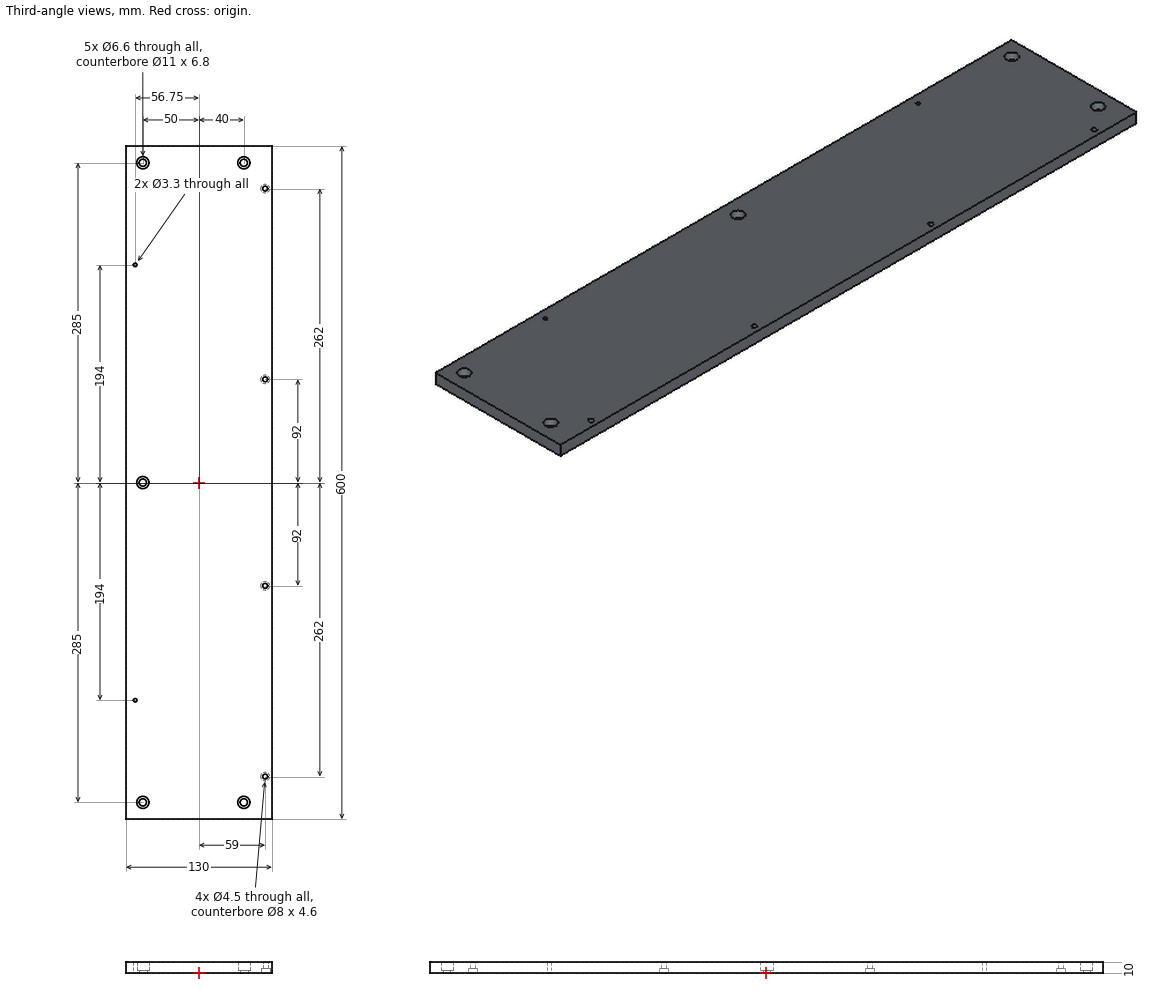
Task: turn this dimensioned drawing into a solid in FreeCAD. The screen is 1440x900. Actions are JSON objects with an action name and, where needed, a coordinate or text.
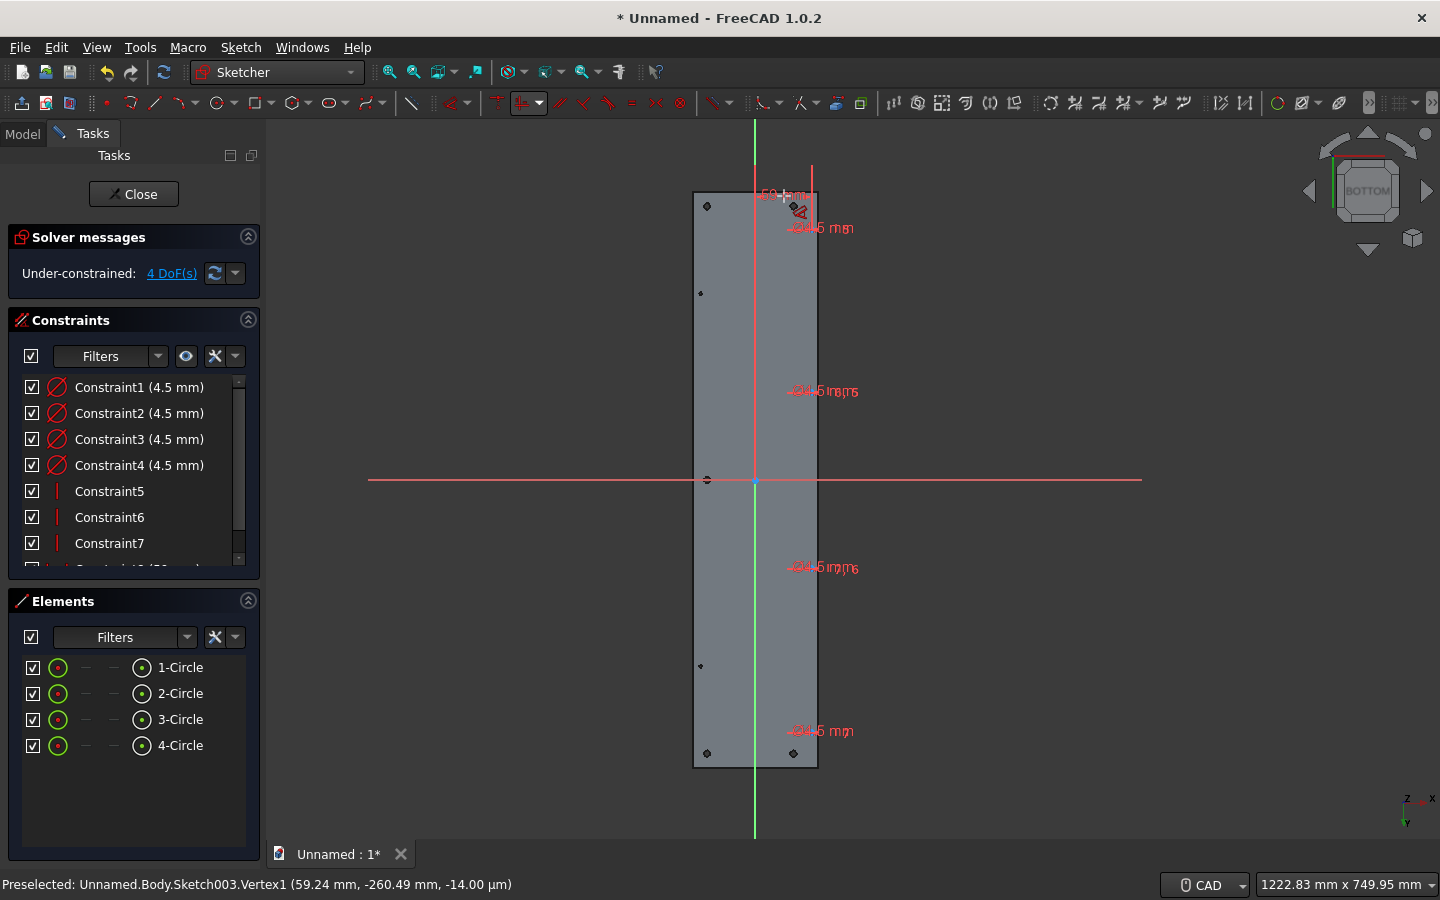
{"action": "left_click", "coordinate": [812, 393]}
{"action": "left_click", "coordinate": [721, 436]}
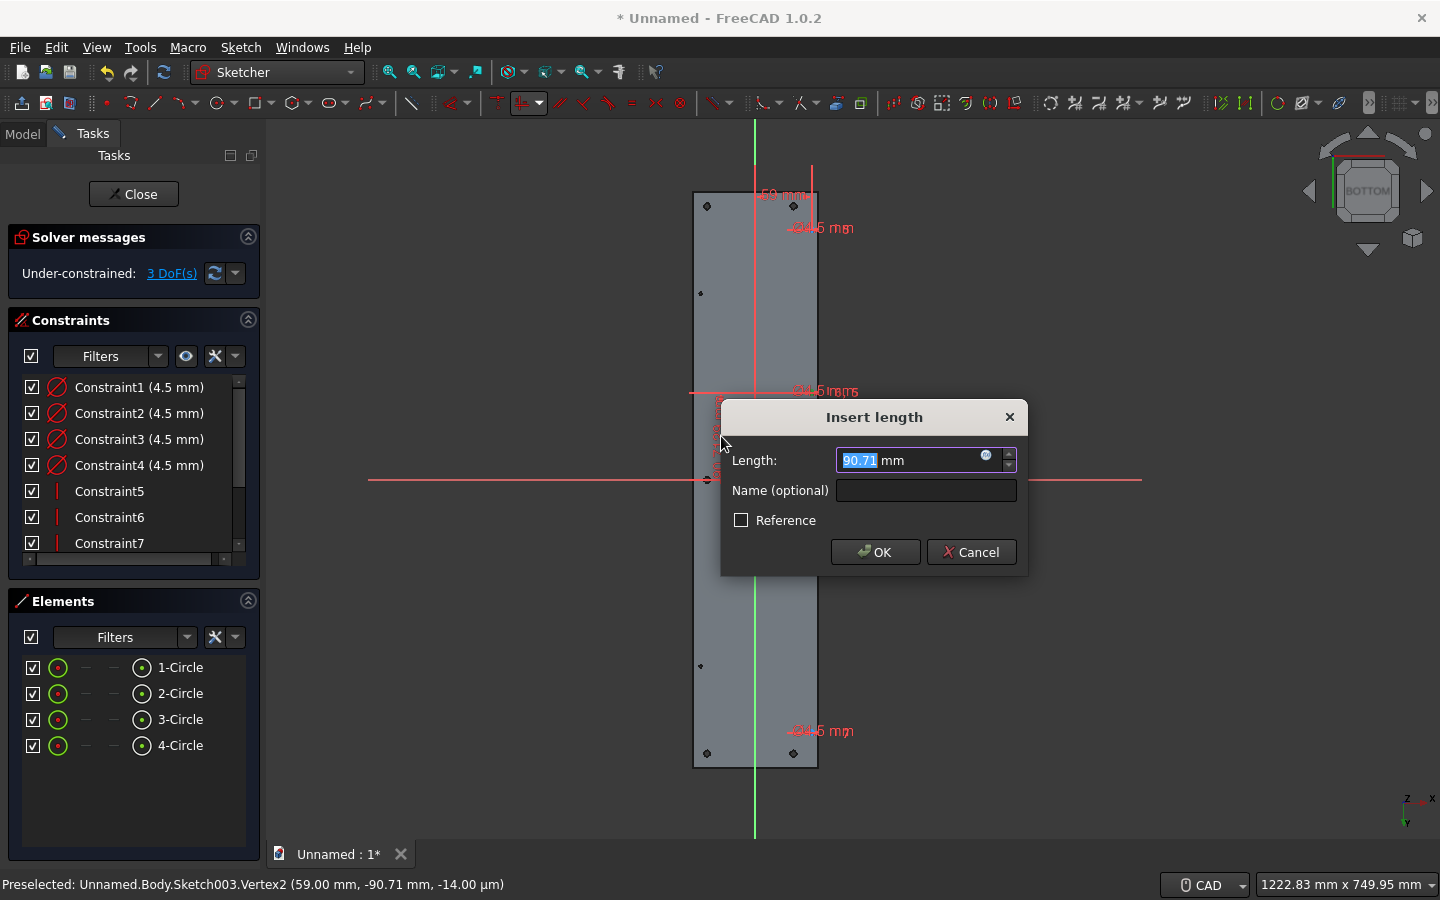
{"action": "type", "text": "92"}
{"action": "key", "text": "Return"}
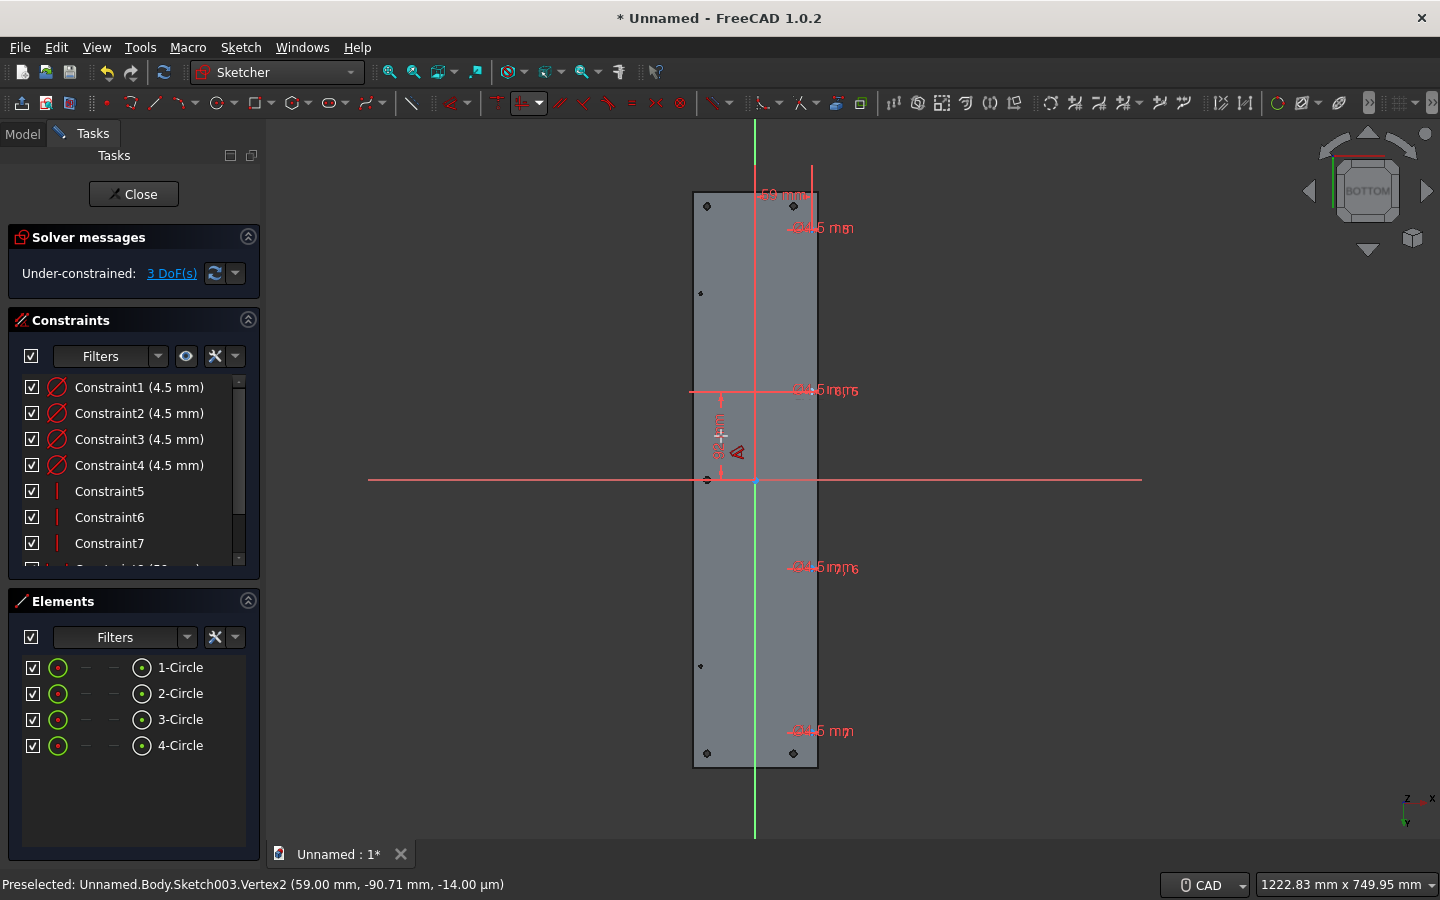
{"action": "left_click", "coordinate": [812, 569]}
{"action": "left_click", "coordinate": [721, 525]}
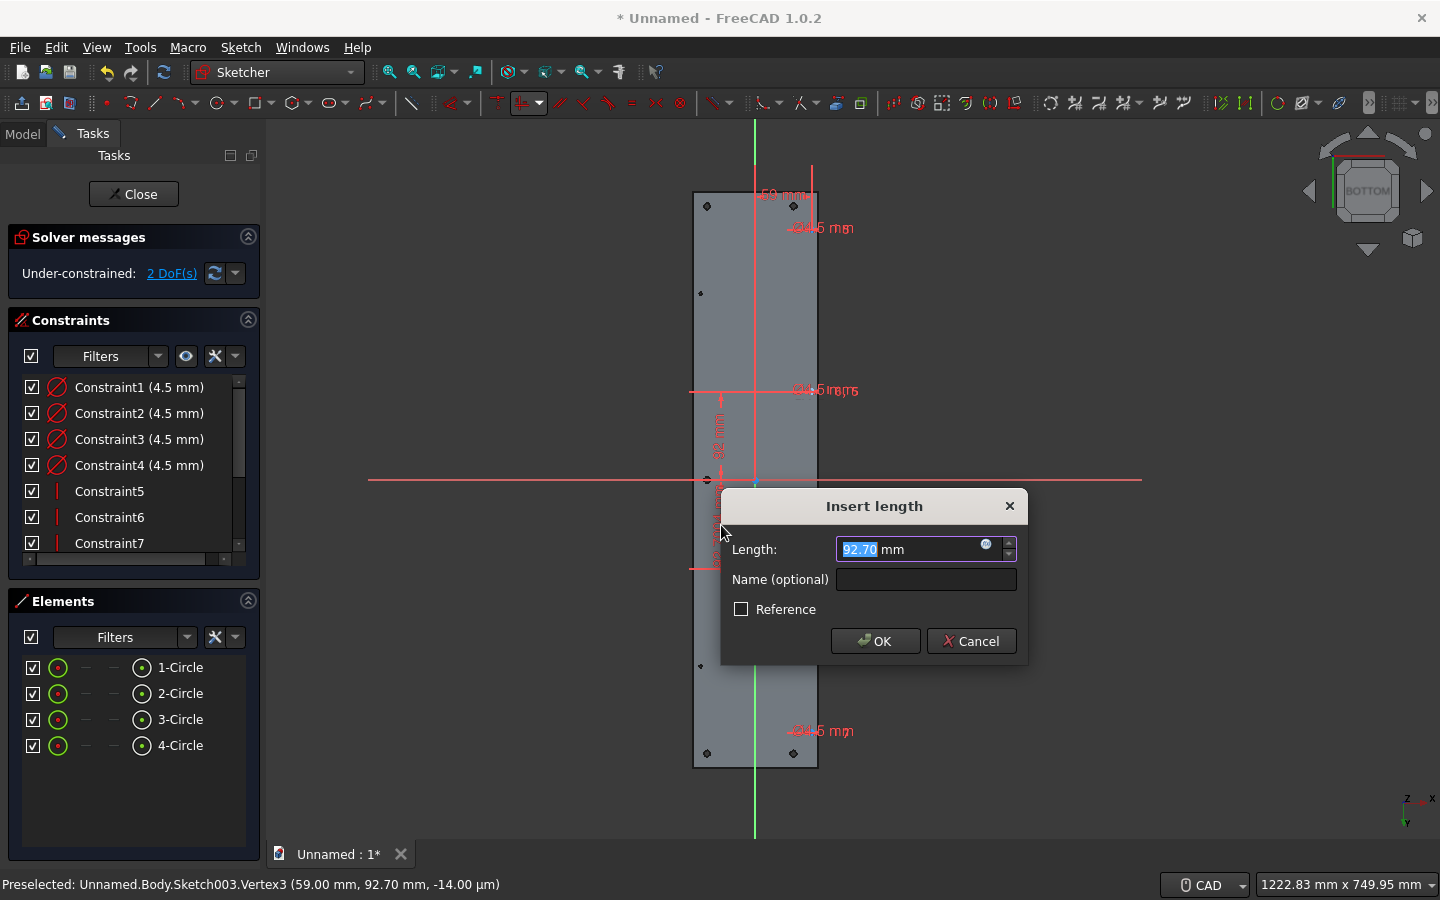
{"action": "type", "text": "92"}
{"action": "key", "text": "Return"}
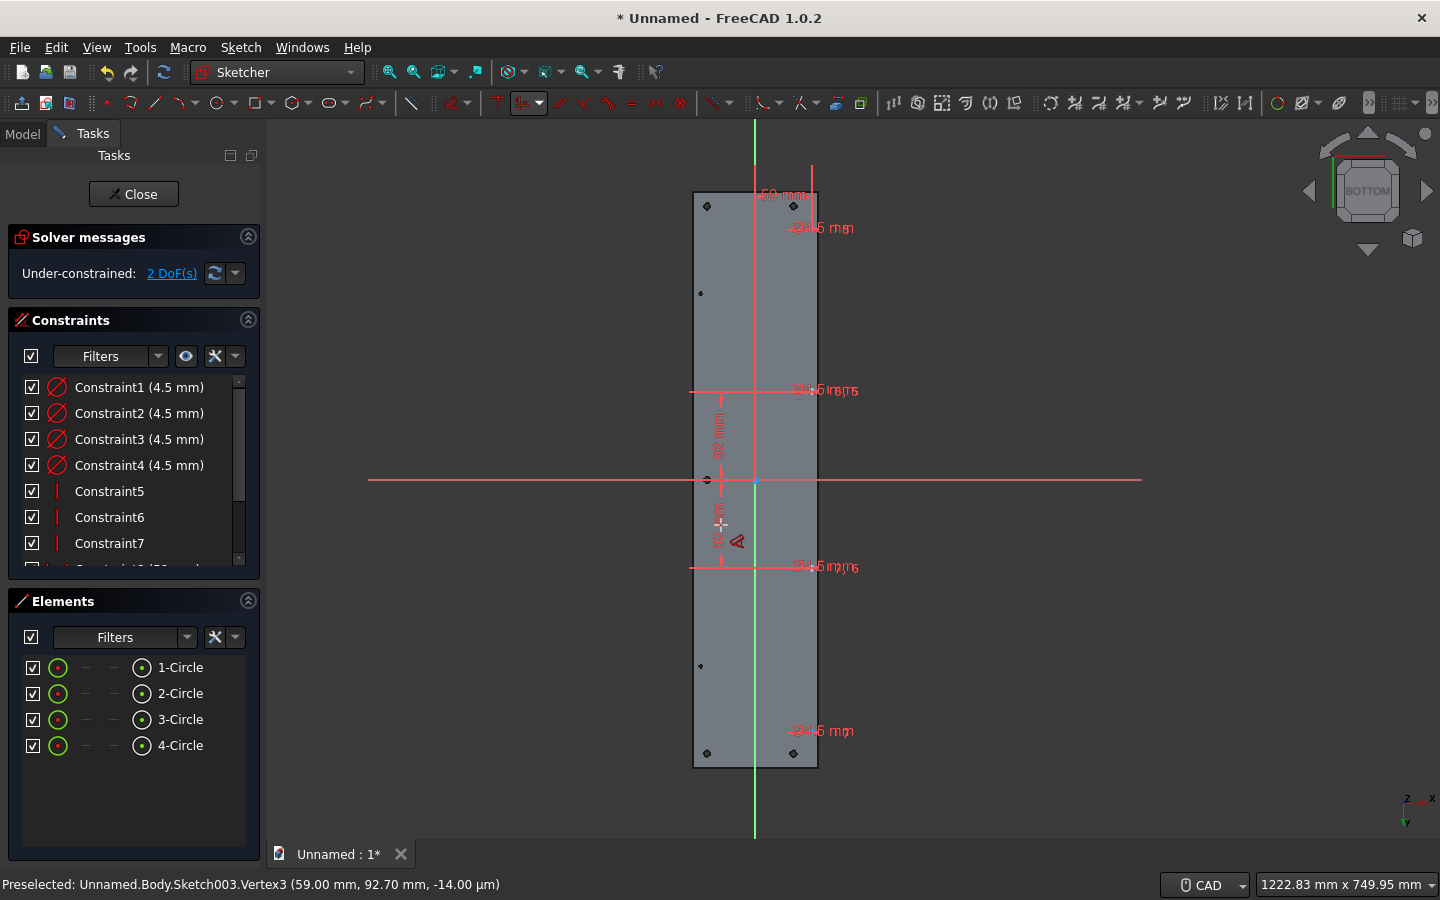
{"action": "left_click", "coordinate": [812, 230]}
{"action": "left_click", "coordinate": [721, 355]}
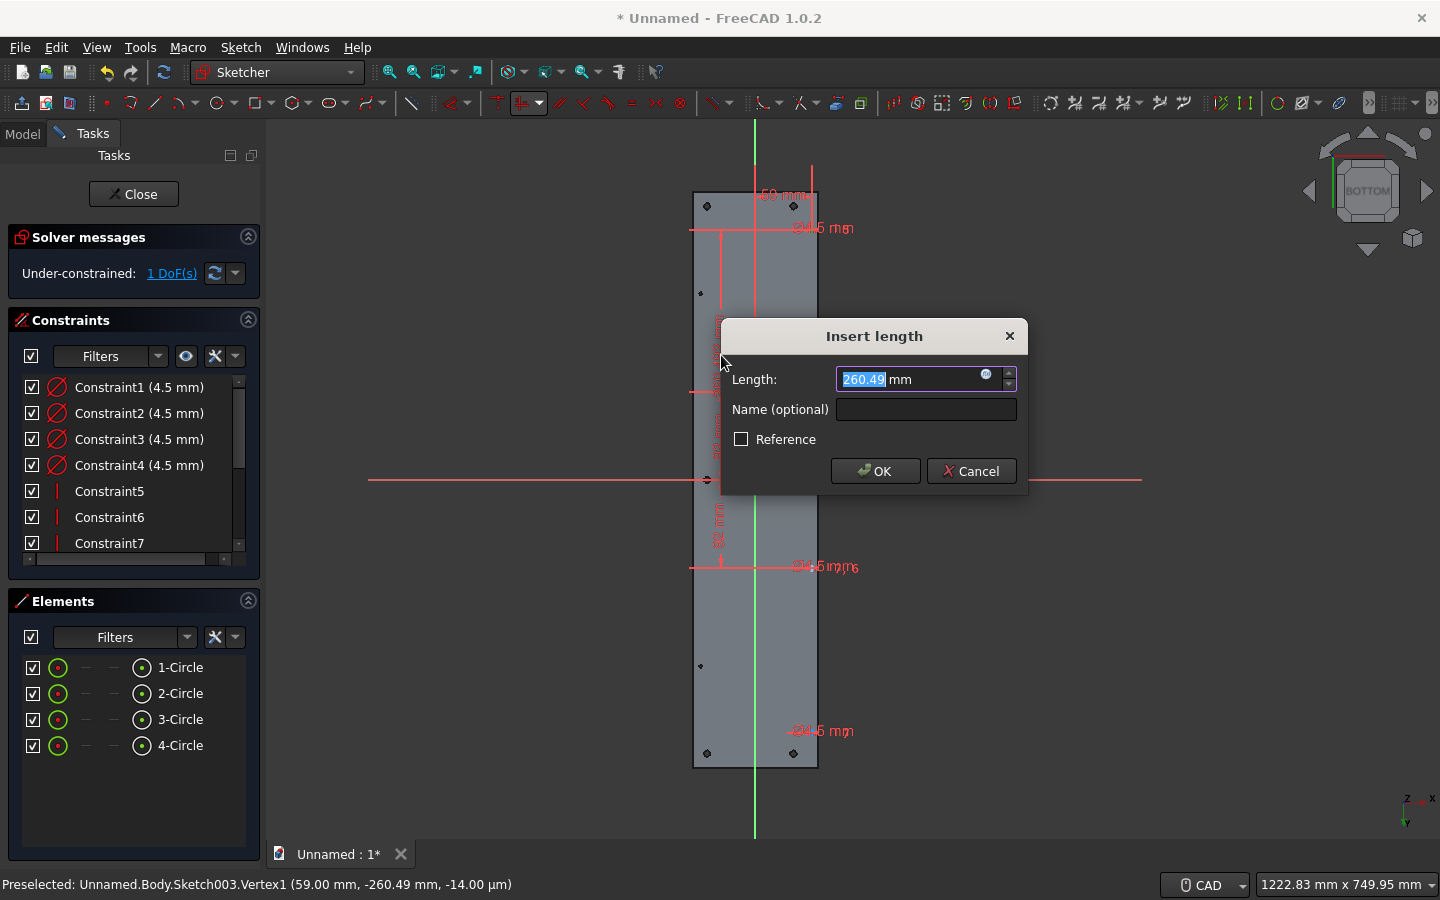
{"action": "type", "text": "262"}
{"action": "key", "text": "Return"}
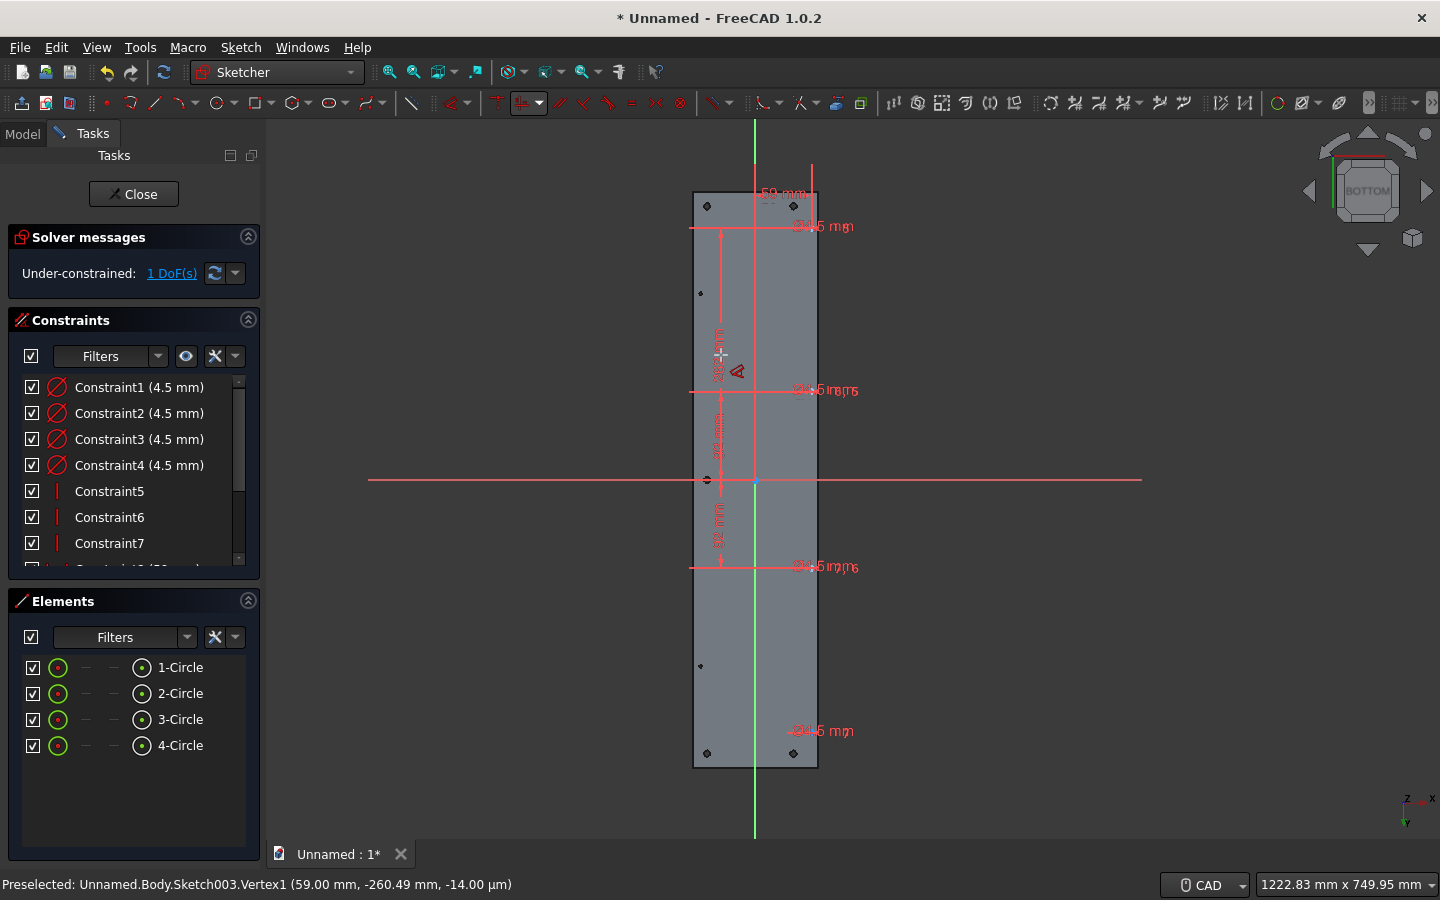
{"action": "left_click", "coordinate": [812, 733]}
{"action": "left_click", "coordinate": [721, 607]}